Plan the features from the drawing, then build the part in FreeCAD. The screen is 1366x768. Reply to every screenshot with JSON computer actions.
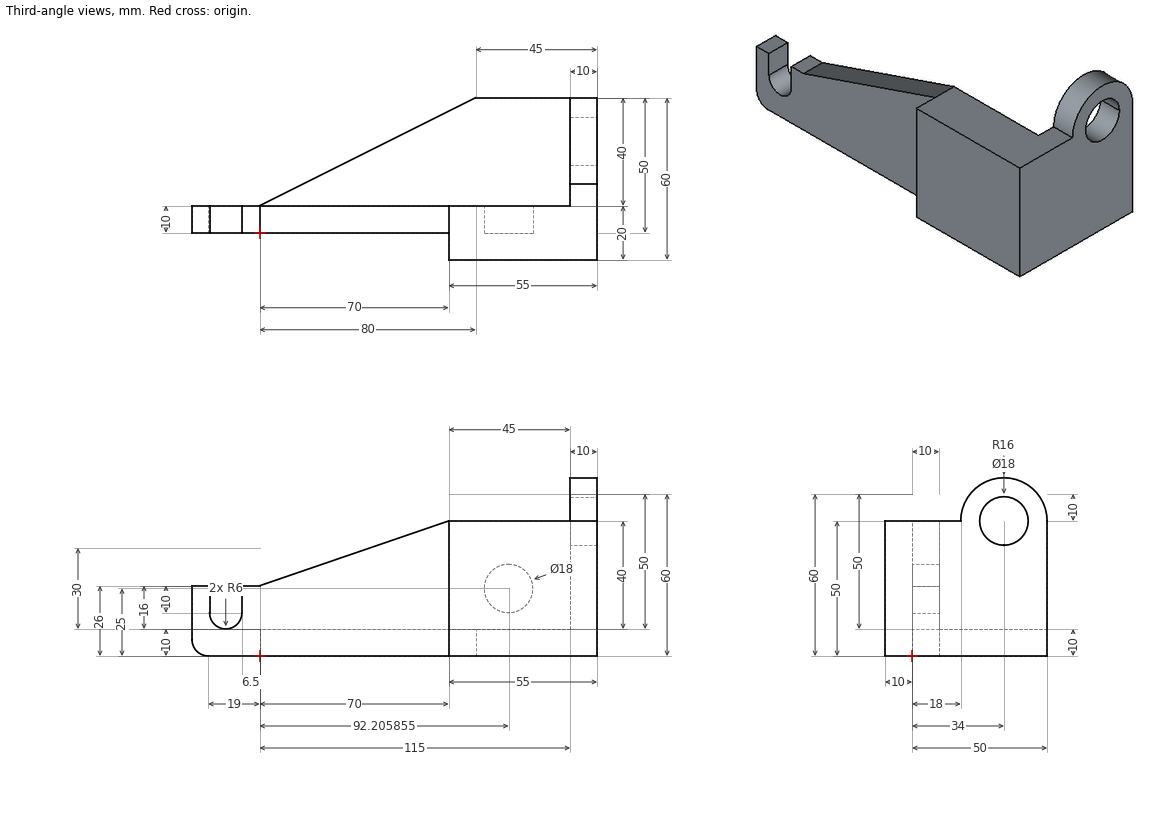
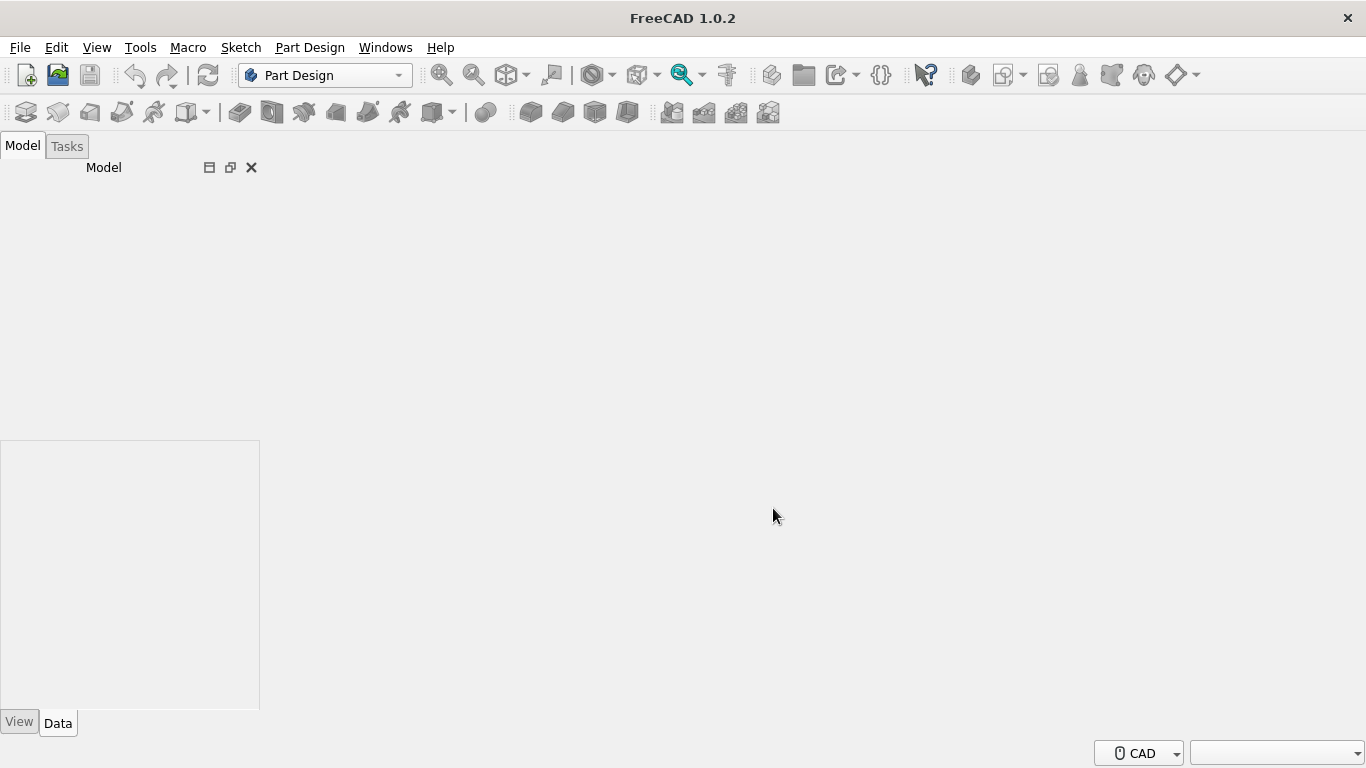
{"action": "left_click", "coordinate": [26, 76]}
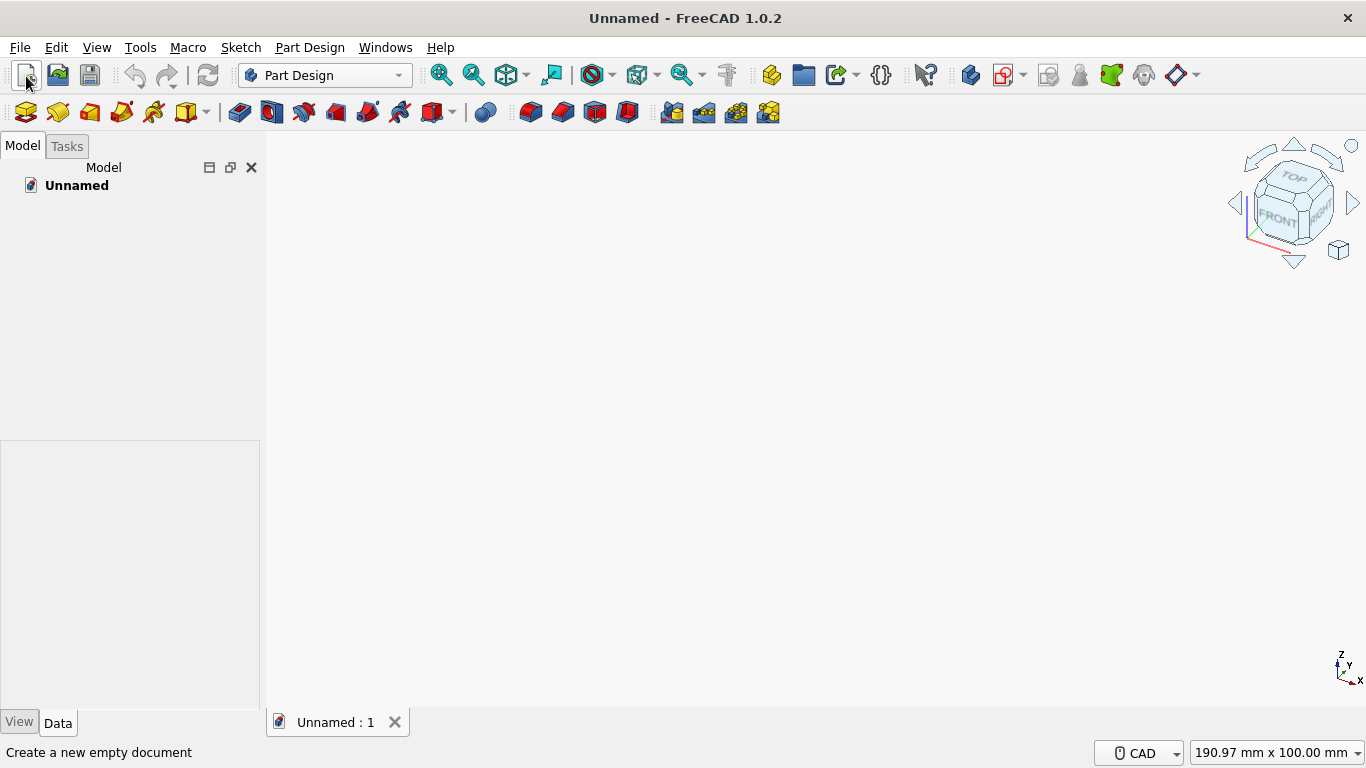
{"action": "left_click", "coordinate": [1004, 76]}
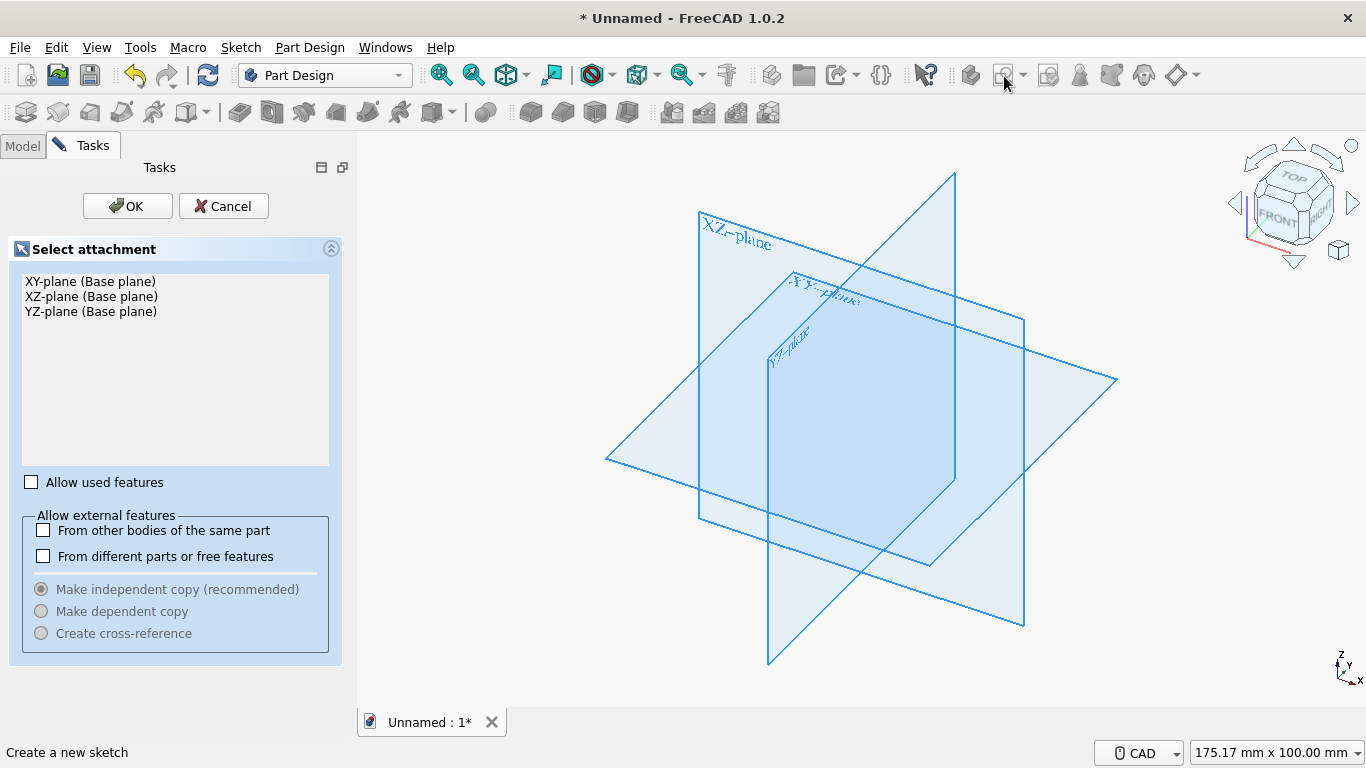
{"action": "left_click", "coordinate": [82, 282]}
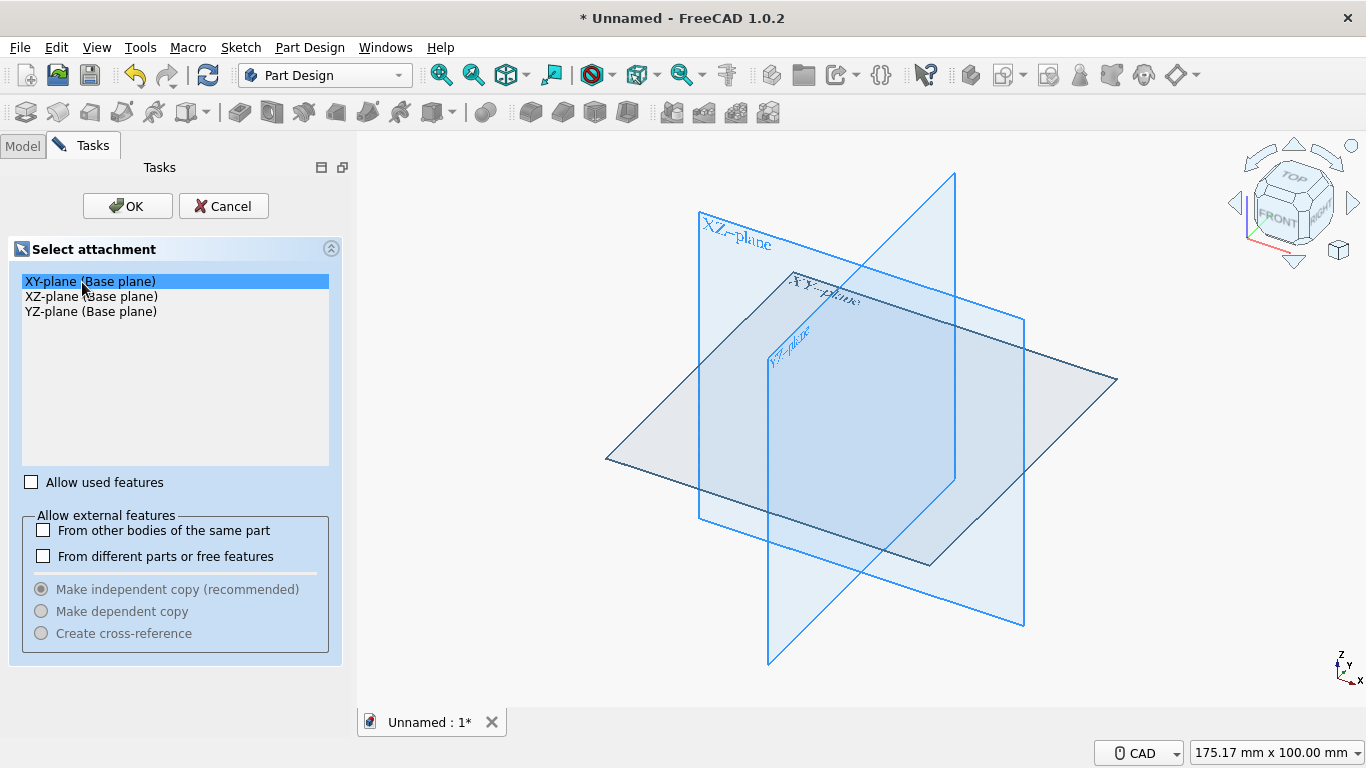
{"action": "left_click", "coordinate": [128, 206]}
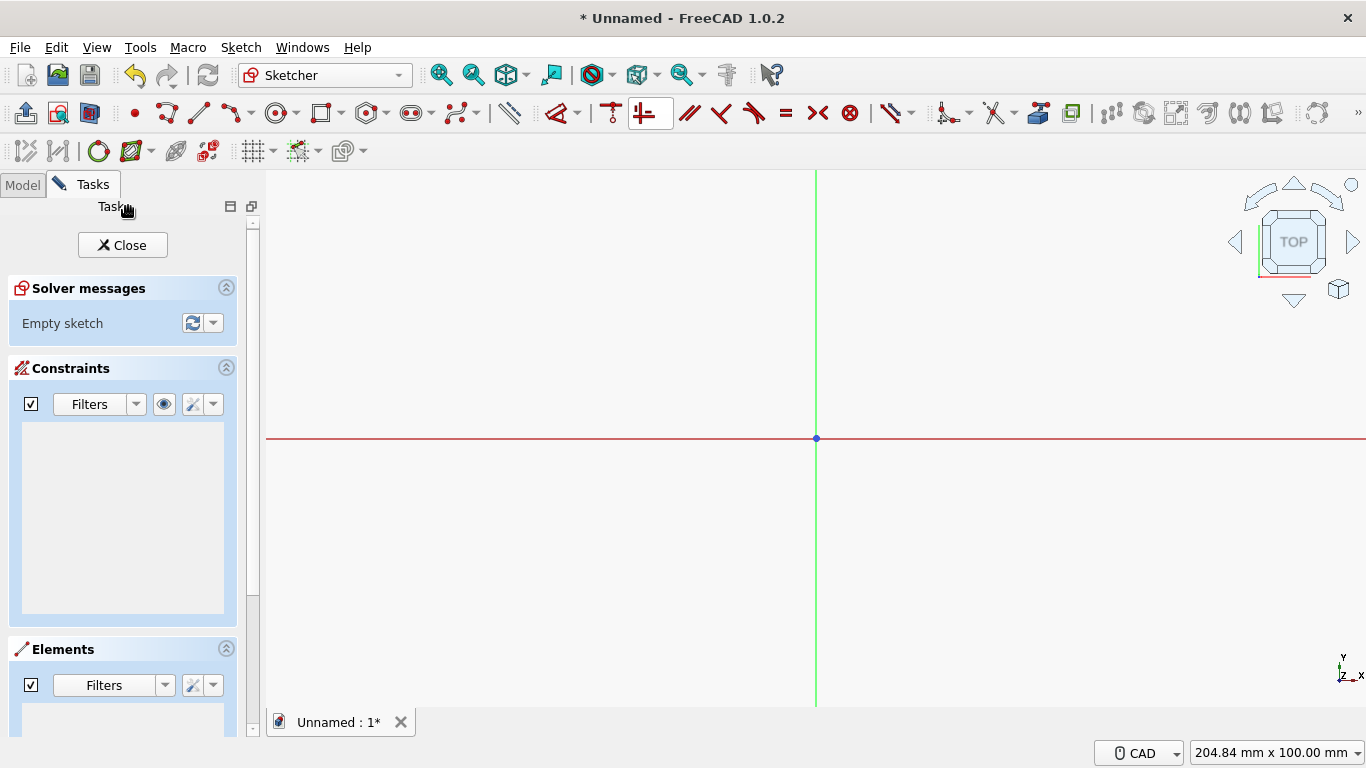
{"action": "scroll", "coordinate": [294, 679], "scroll_direction": "down", "scroll_amount": 2}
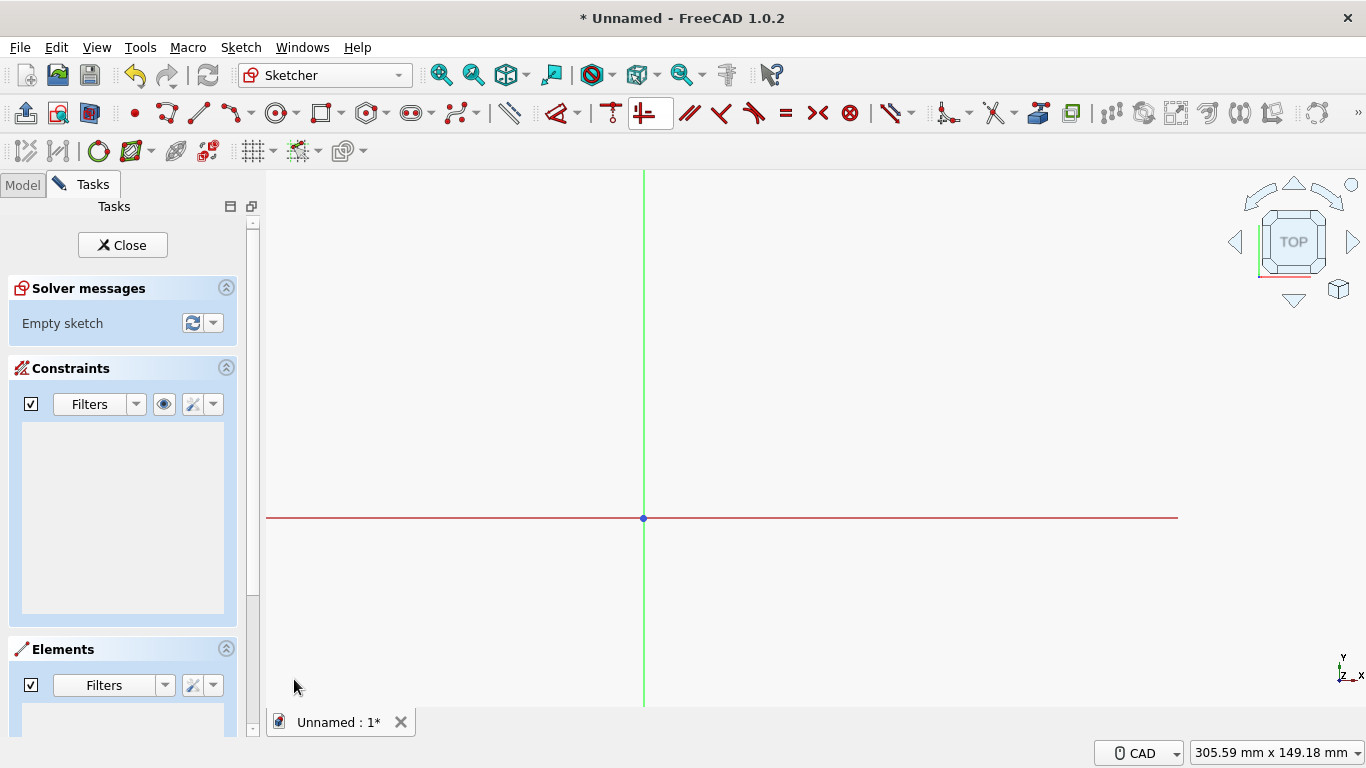
{"action": "scroll", "coordinate": [1116, 407], "scroll_direction": "up", "scroll_amount": 2}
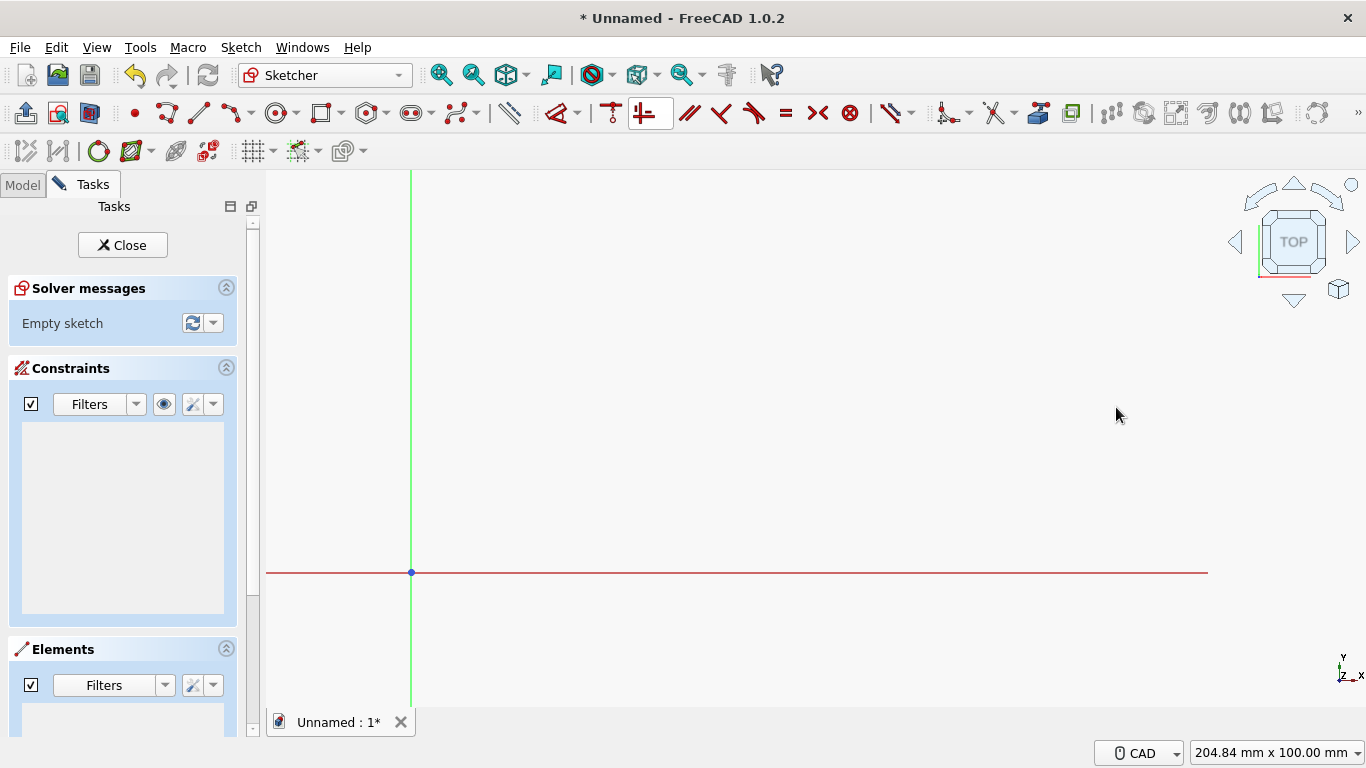
{"action": "left_click", "coordinate": [168, 114]}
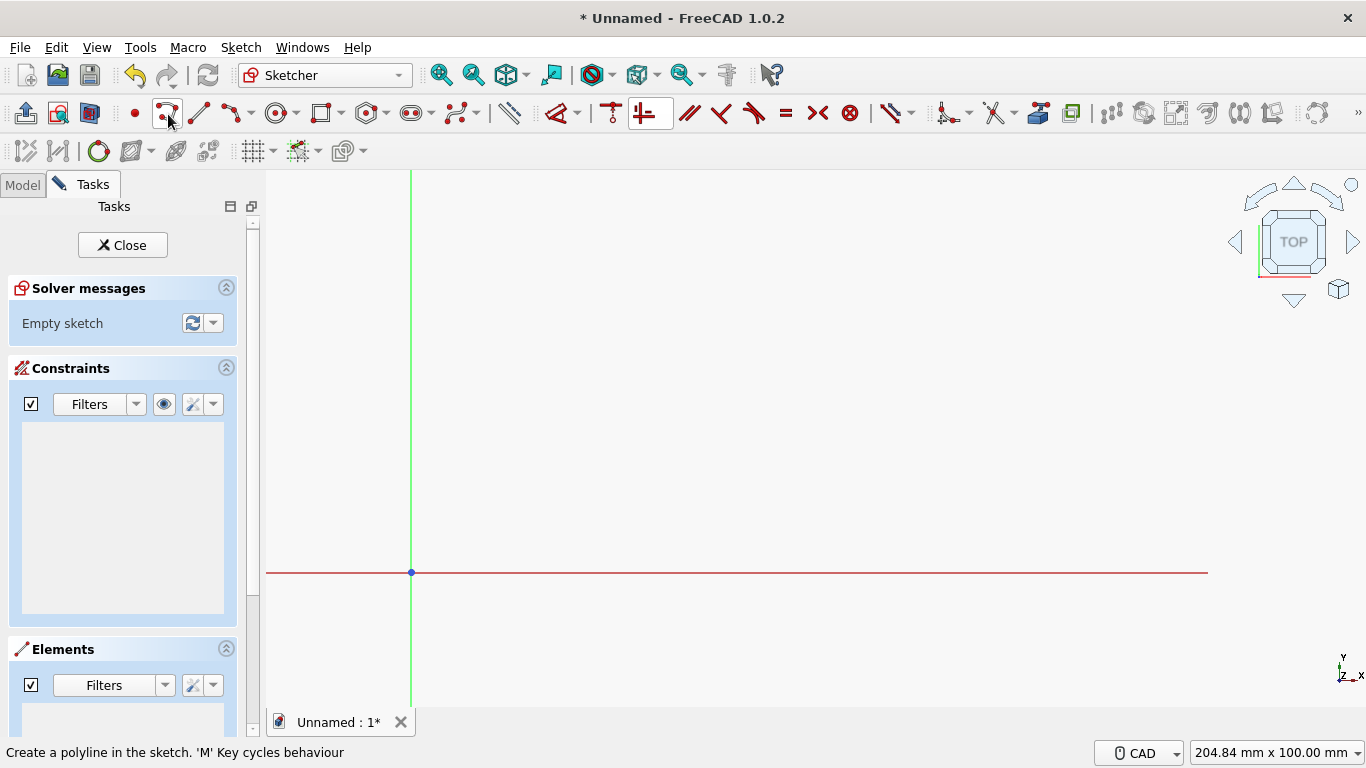
{"action": "left_click", "coordinate": [411, 573]}
{"action": "left_click", "coordinate": [1083, 564]}
{"action": "left_click", "coordinate": [1083, 304]}
{"action": "left_click", "coordinate": [841, 304]}
{"action": "left_click", "coordinate": [841, 519]}
{"action": "left_click", "coordinate": [420, 519]}
{"action": "left_click", "coordinate": [411, 573]}
{"action": "key", "text": "Escape"}
{"action": "key", "text": "Escape"}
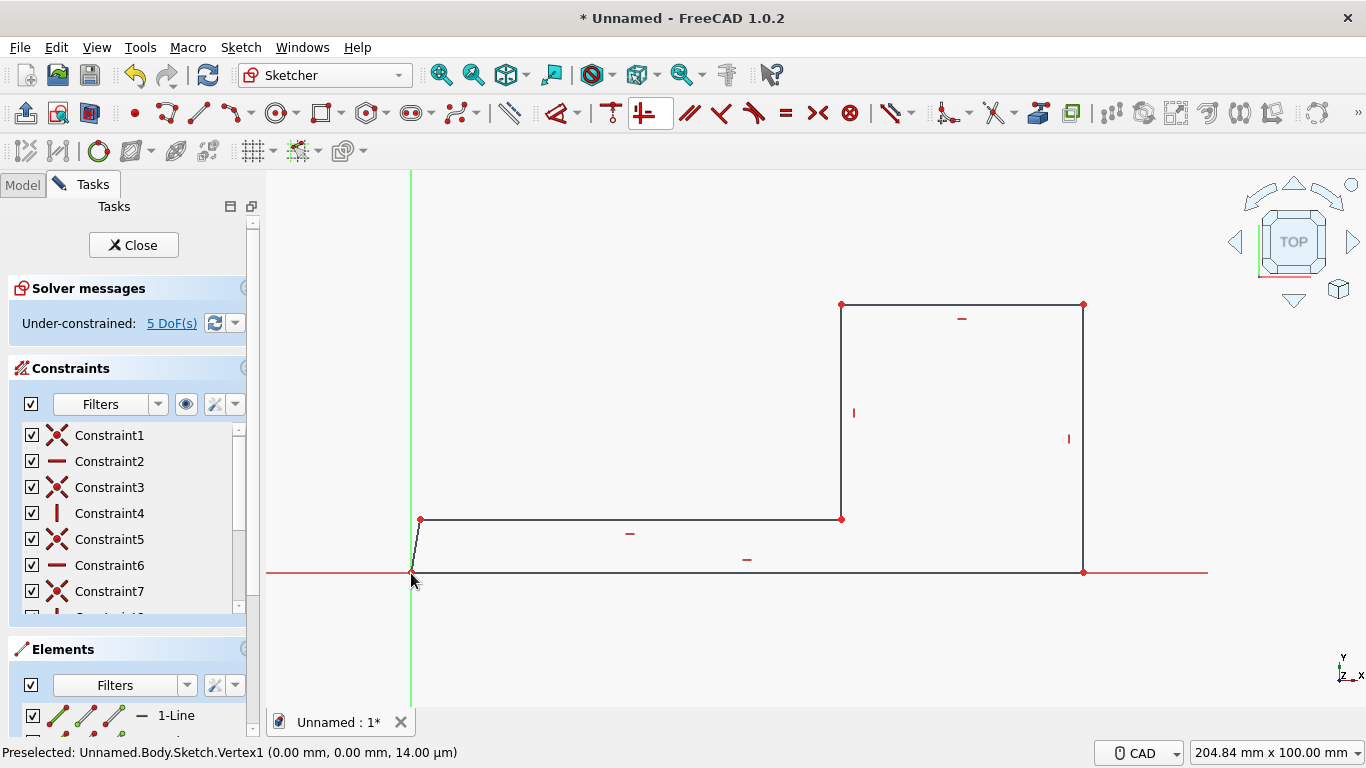
{"action": "left_click", "coordinate": [414, 557]}